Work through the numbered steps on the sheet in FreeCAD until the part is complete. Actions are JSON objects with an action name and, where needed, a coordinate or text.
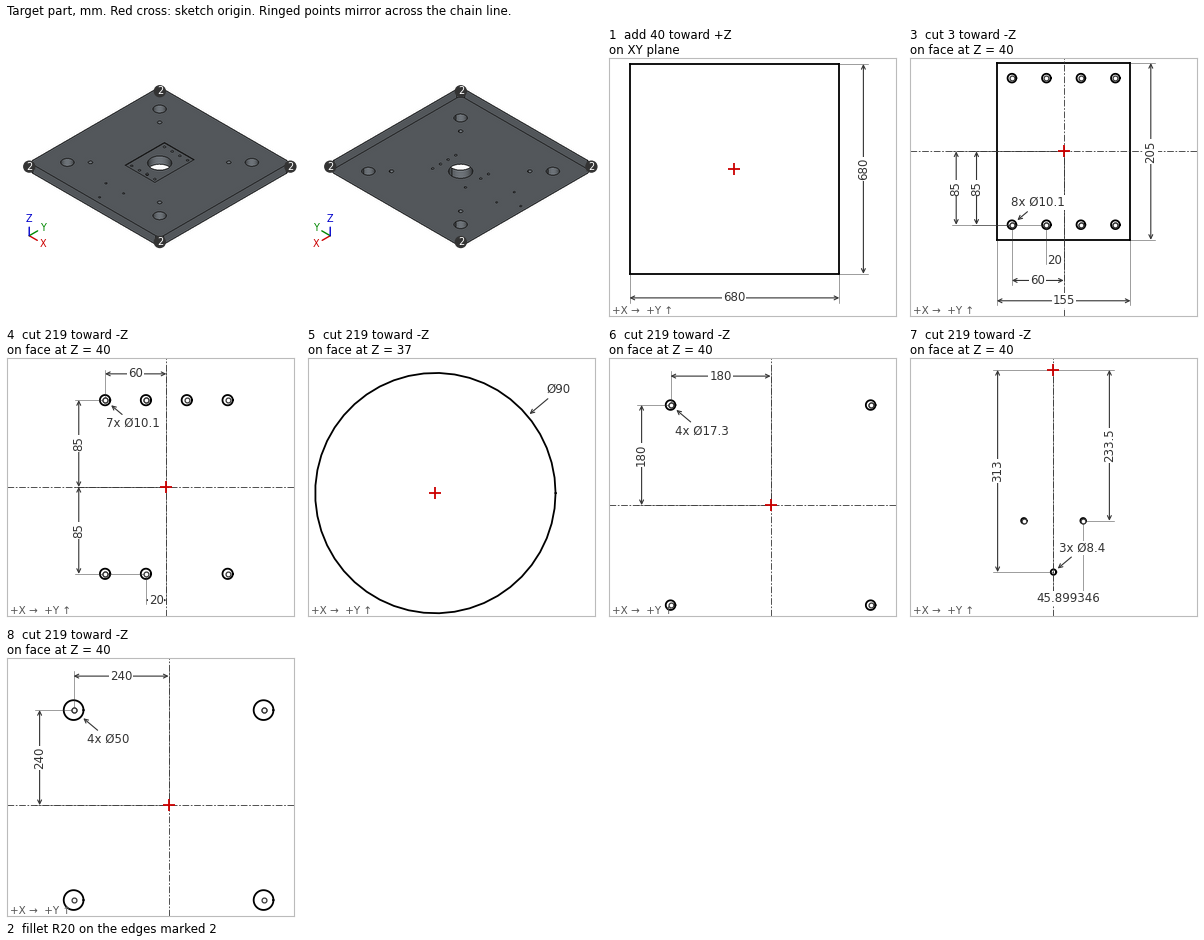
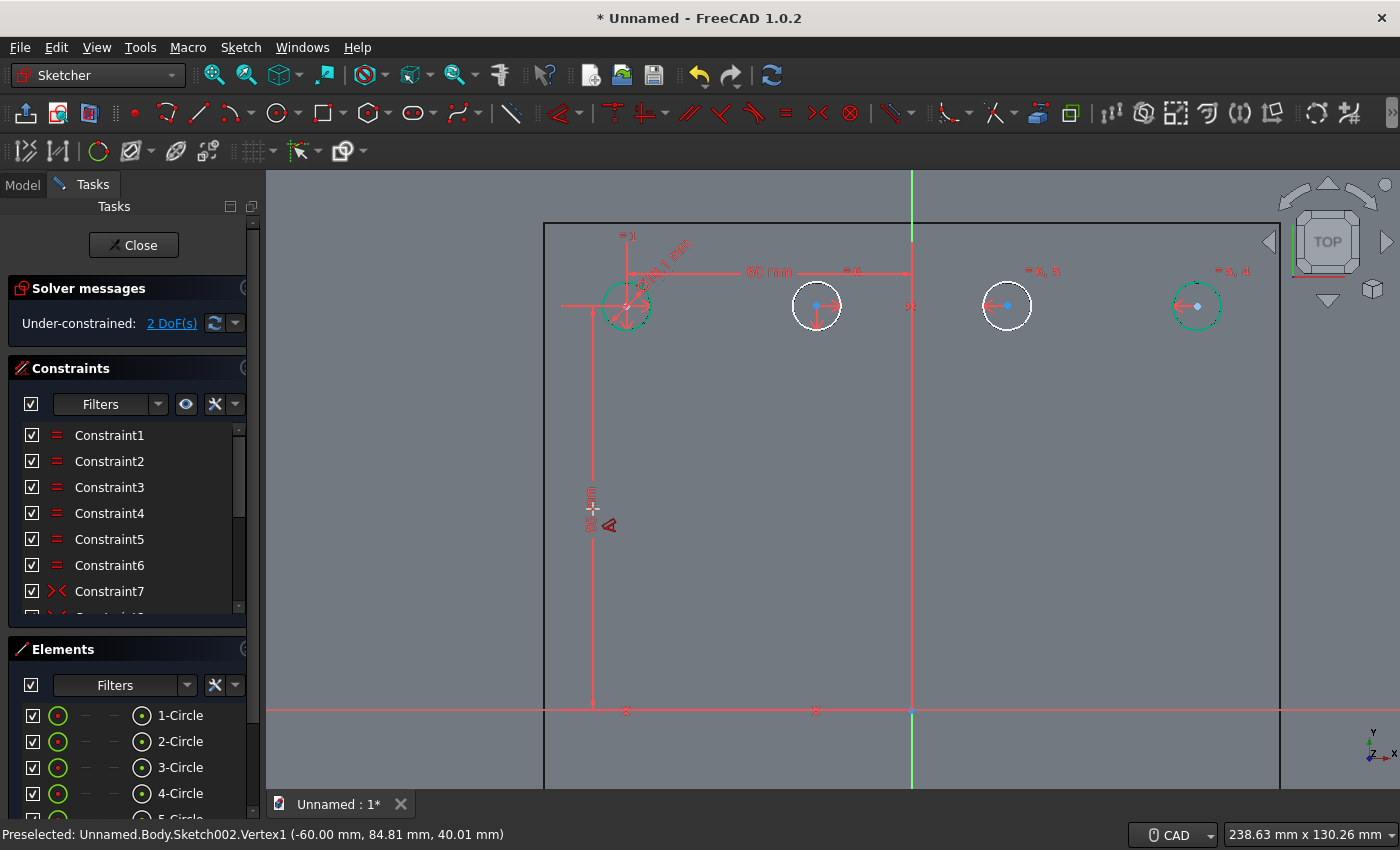
{"action": "scroll", "coordinate": [644, 291], "scroll_direction": "down", "scroll_amount": 4}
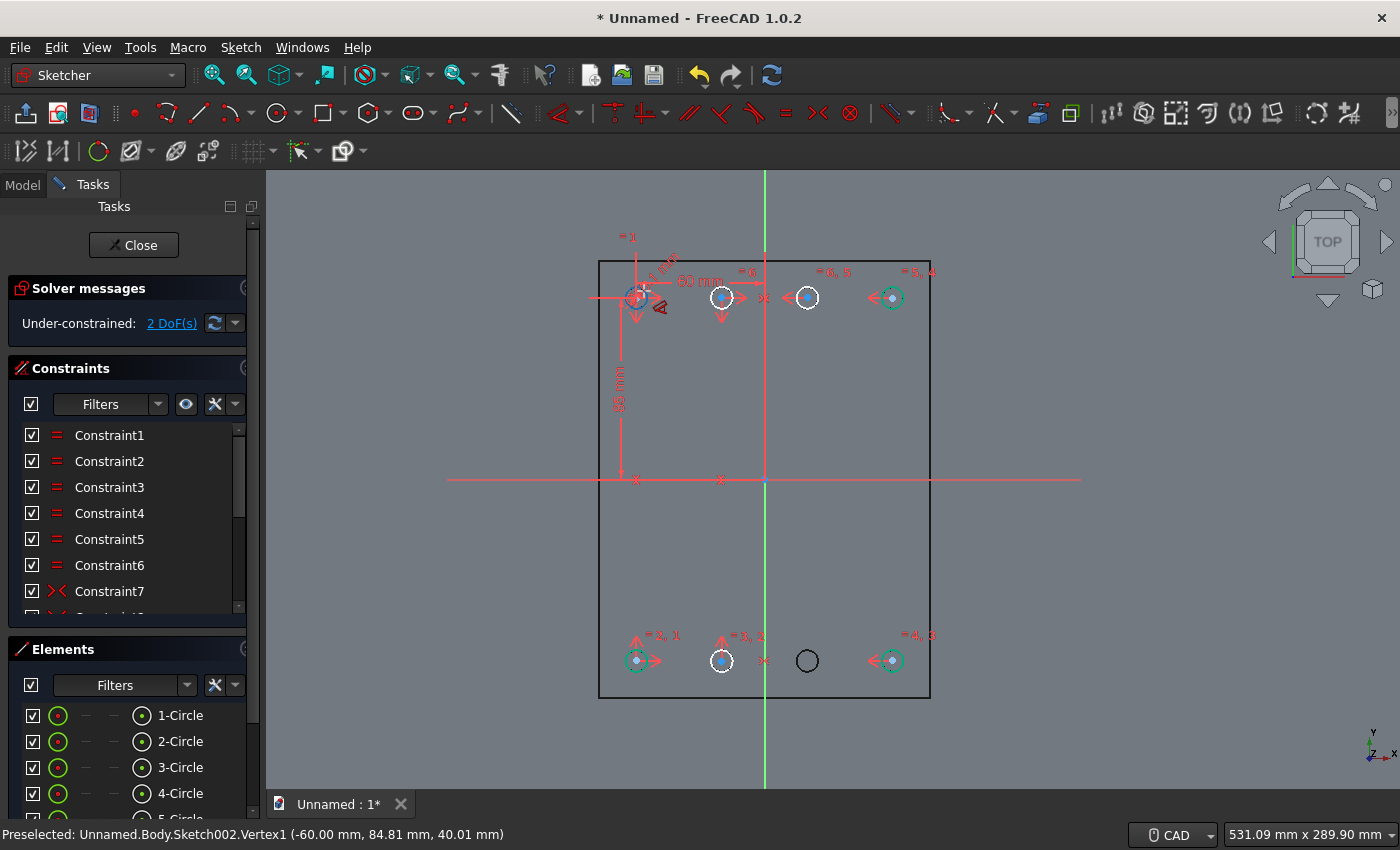
{"action": "left_click", "coordinate": [722, 661]}
{"action": "left_click", "coordinate": [743, 695]}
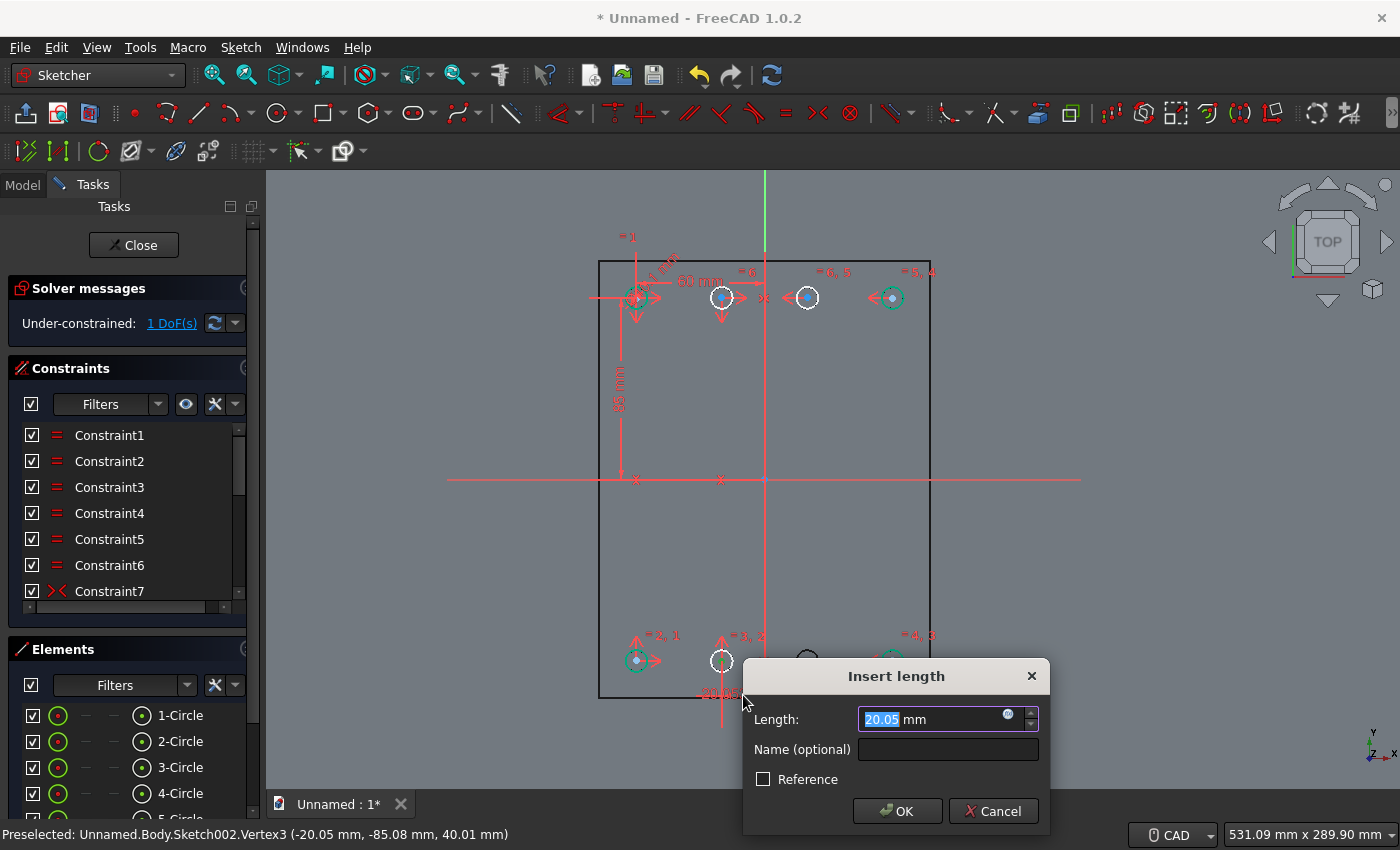
{"action": "type", "text": "20"}
{"action": "key", "text": "Return"}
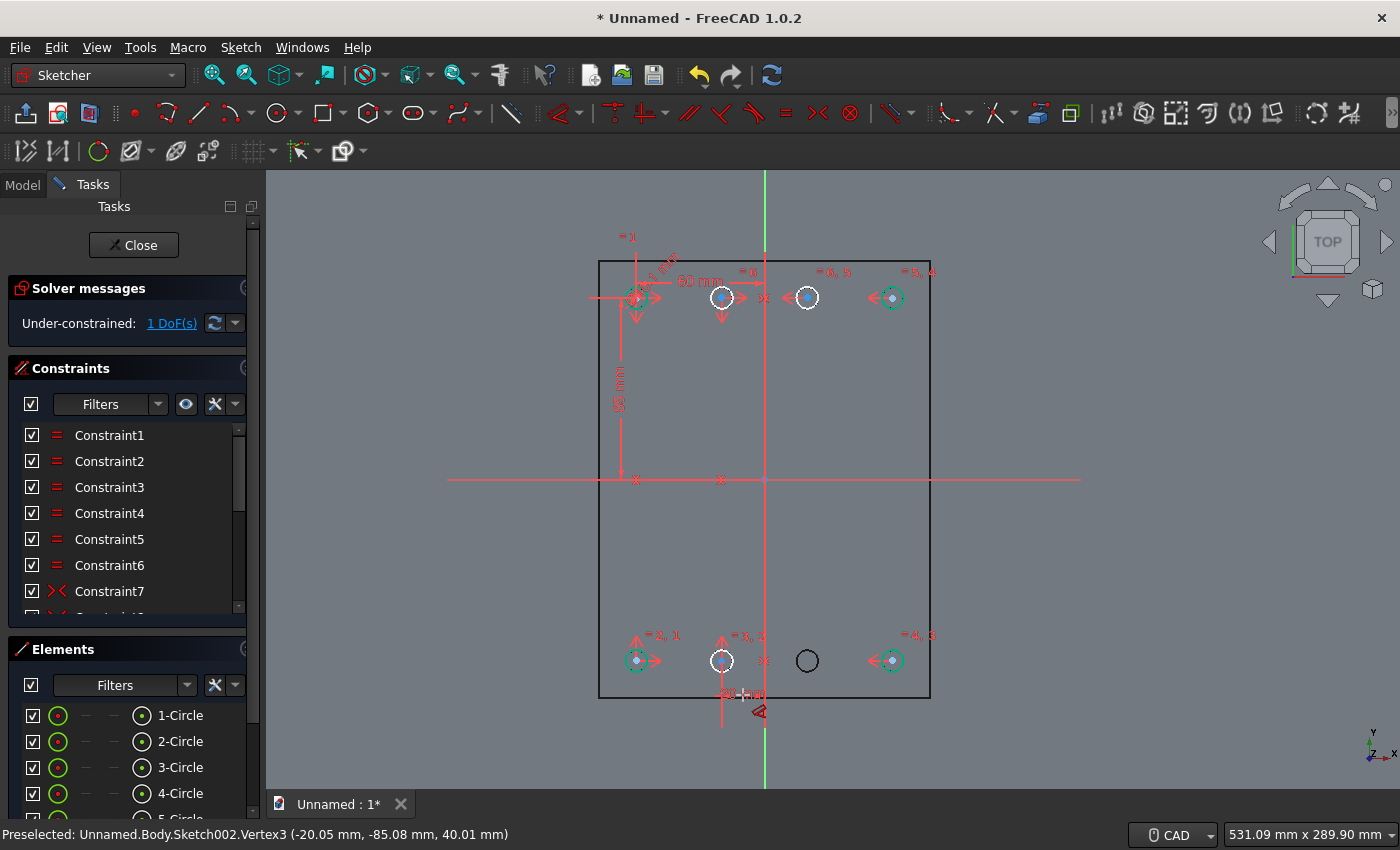
{"action": "left_click", "coordinate": [722, 661]}
{"action": "left_click", "coordinate": [688, 570]}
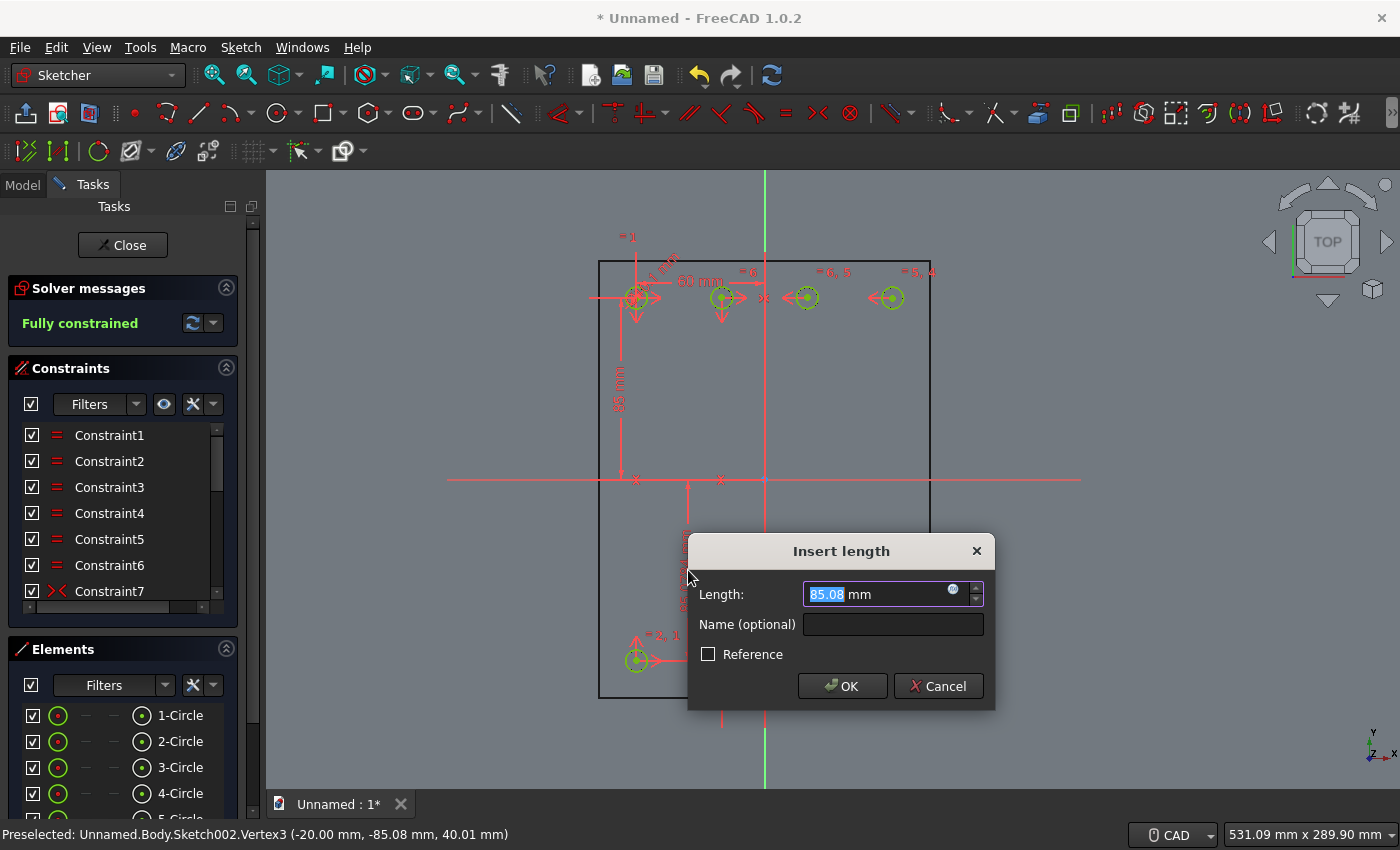
{"action": "type", "text": "85"}
{"action": "key", "text": "Return"}
{"action": "key", "text": "Escape"}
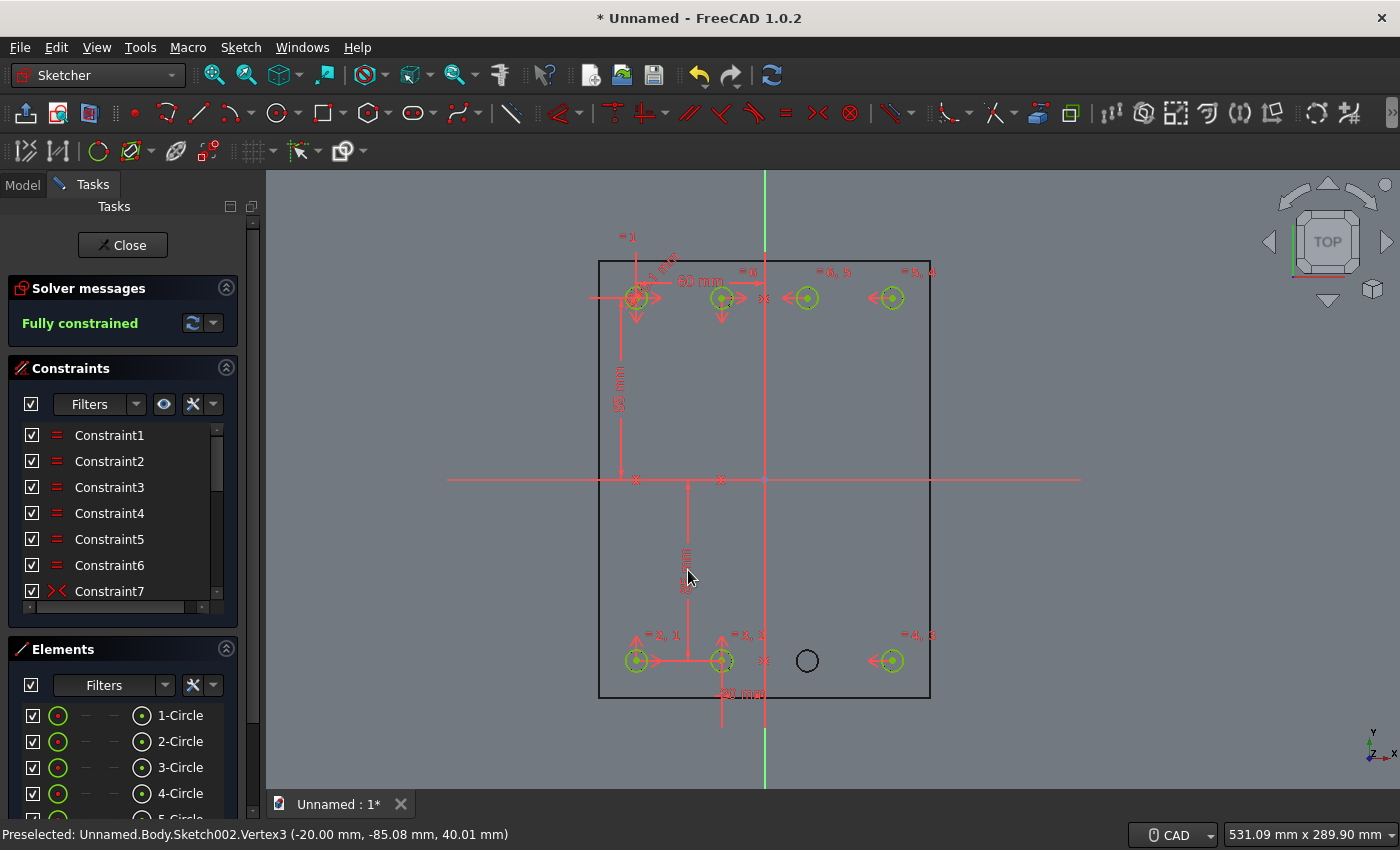
{"action": "left_click", "coordinate": [123, 245]}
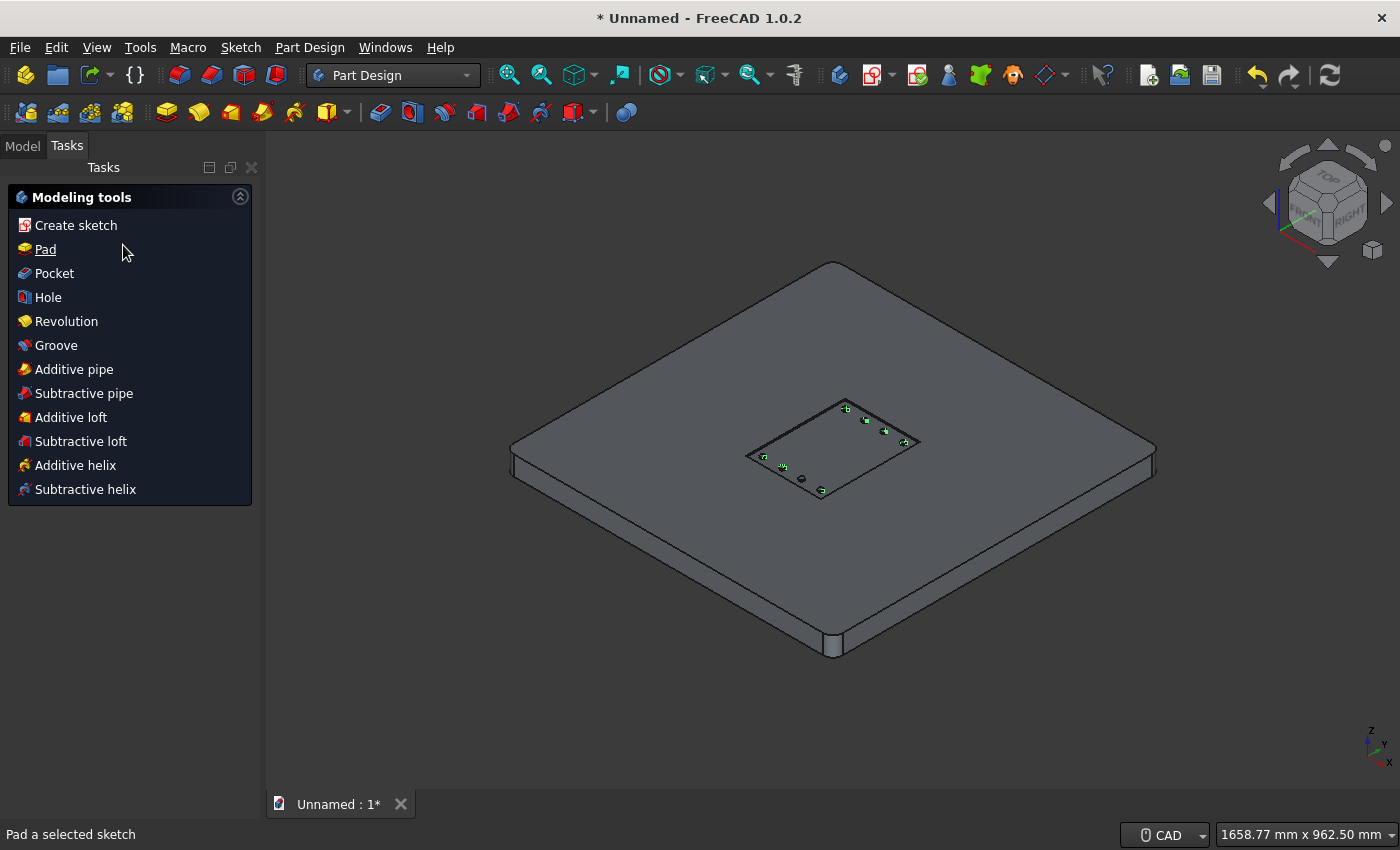
{"action": "left_click", "coordinate": [382, 112]}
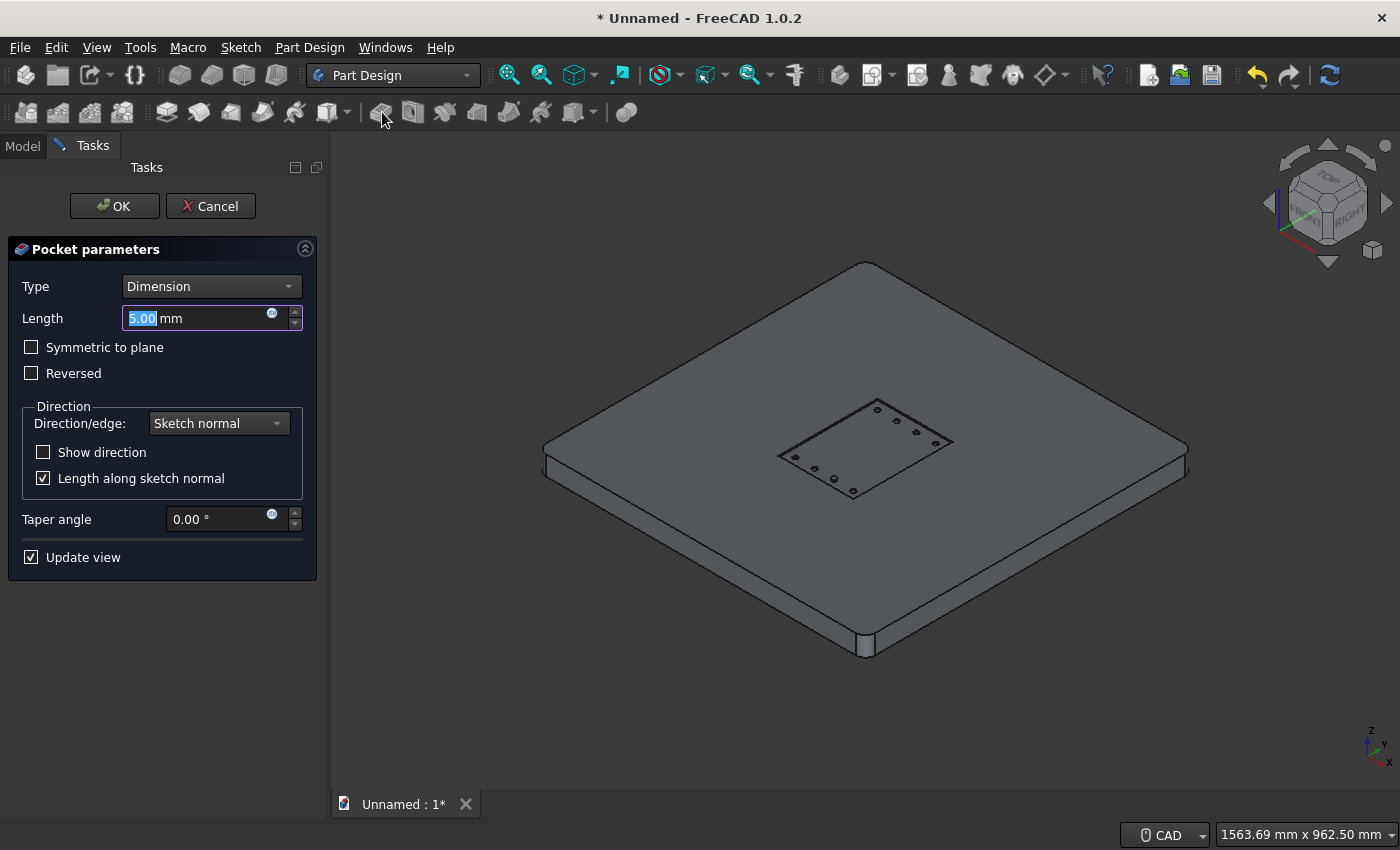
{"action": "type", "text": "219"}
{"action": "key", "text": "Tab"}